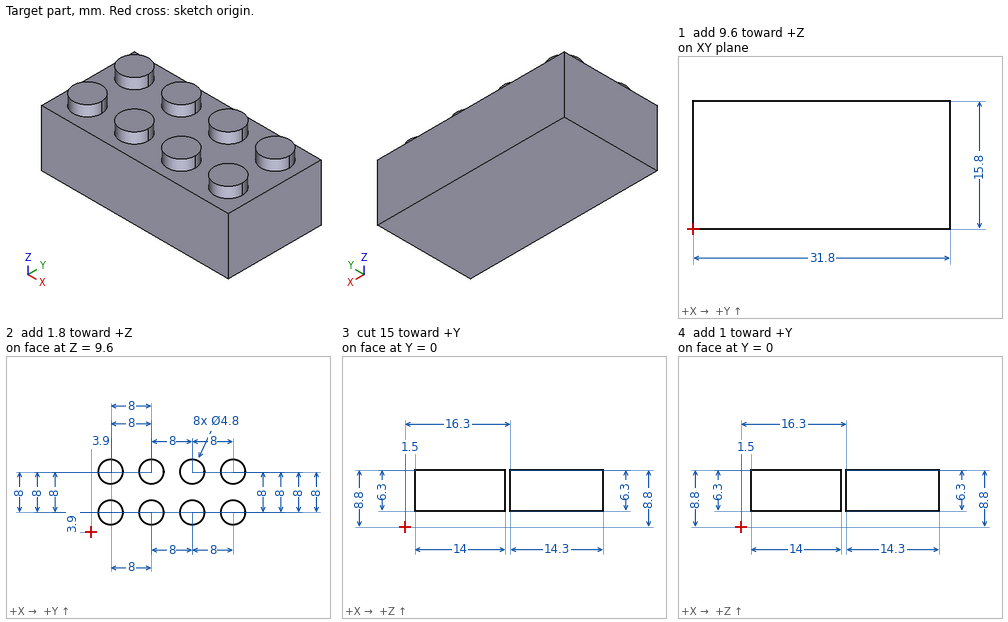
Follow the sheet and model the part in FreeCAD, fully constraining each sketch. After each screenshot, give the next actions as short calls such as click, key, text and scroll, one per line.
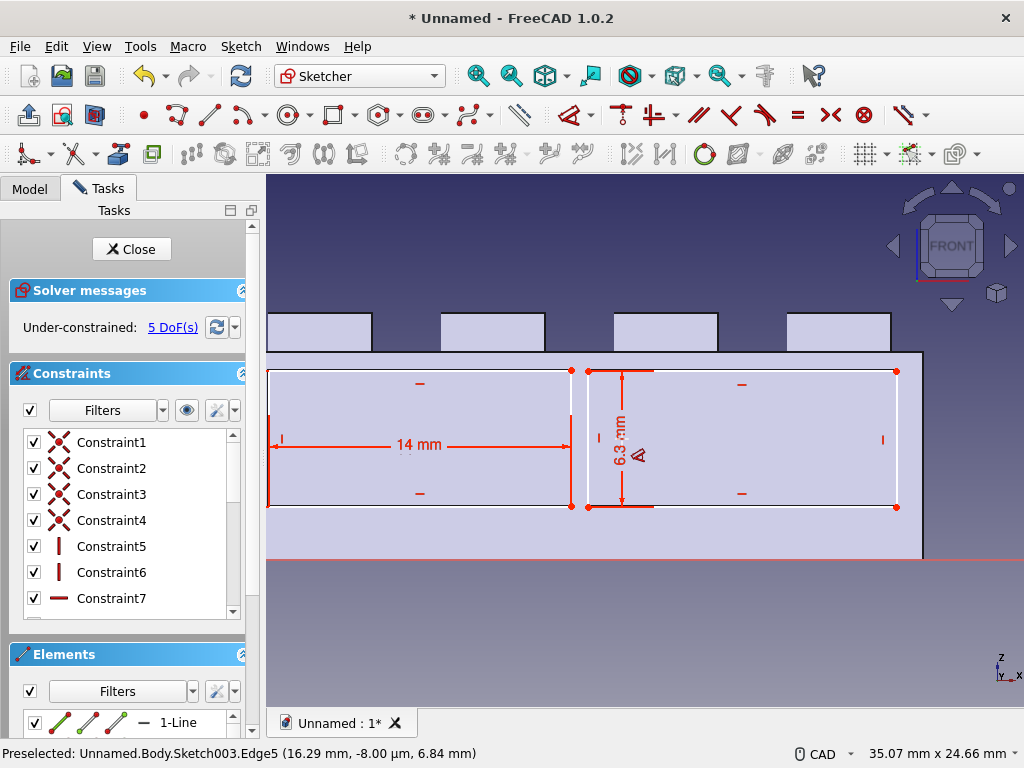
click(681, 507)
click(724, 541)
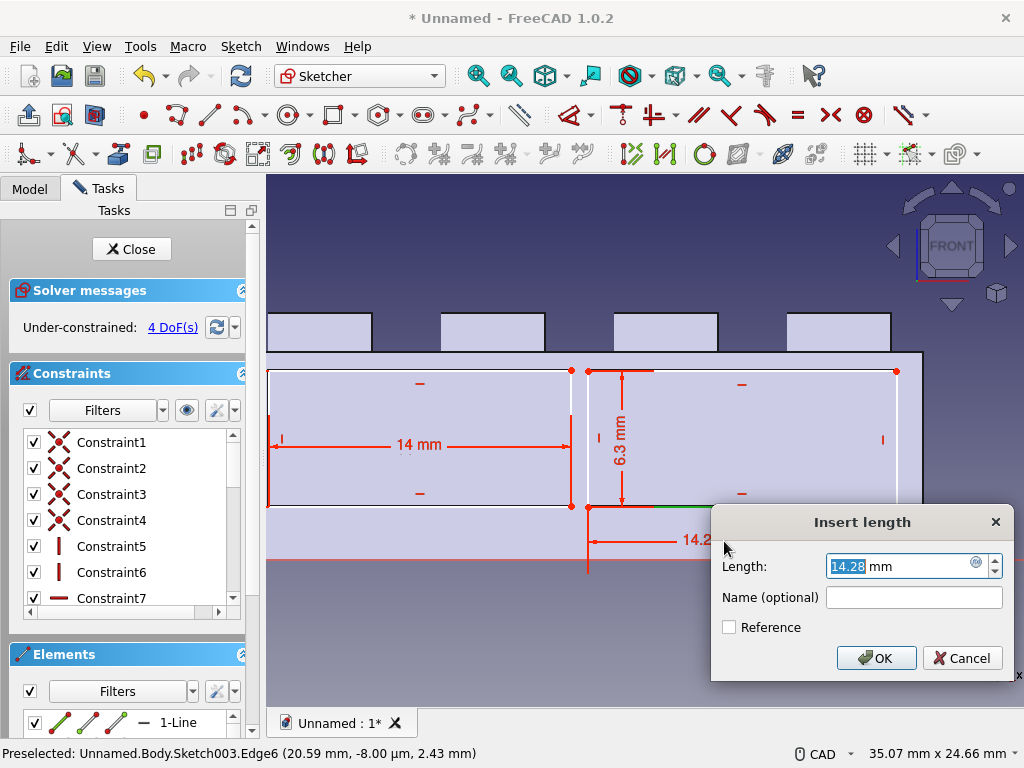
text(14.3)
key(Return)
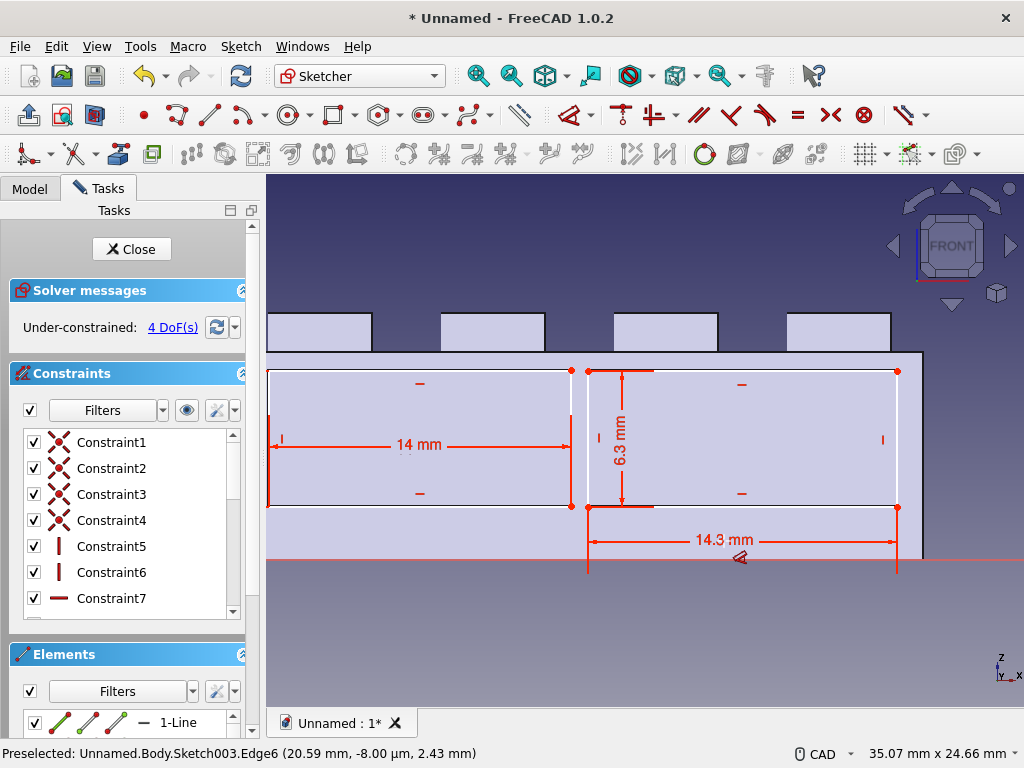
scroll(589, 411, down, 3)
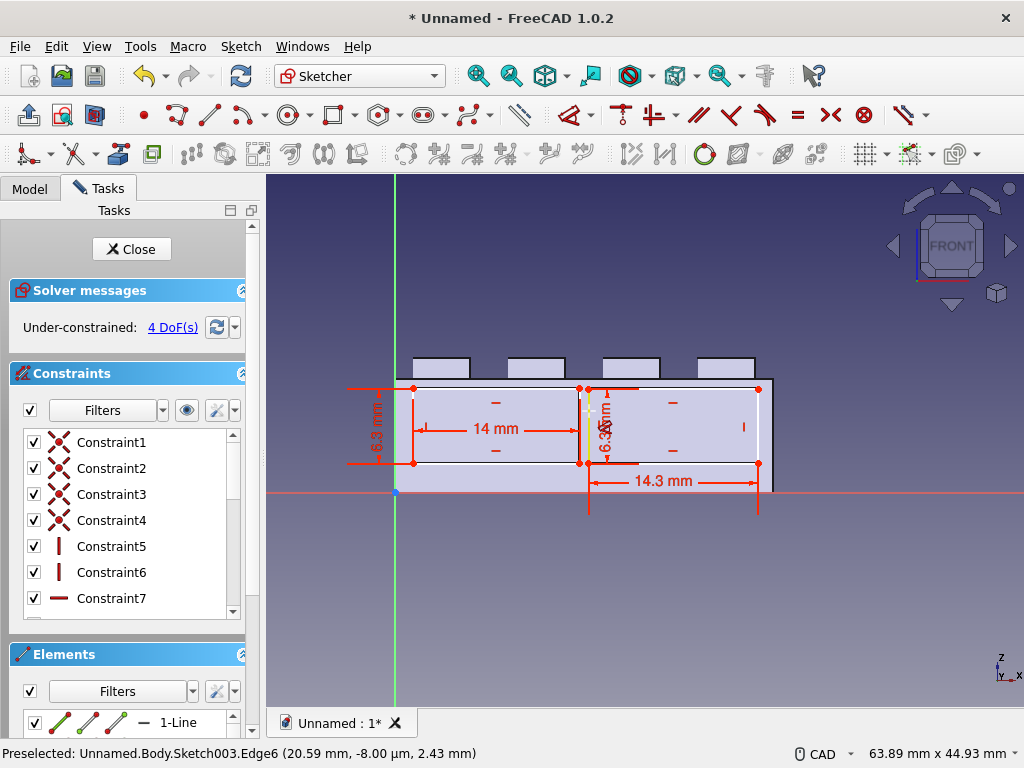
scroll(413, 389, up, 5)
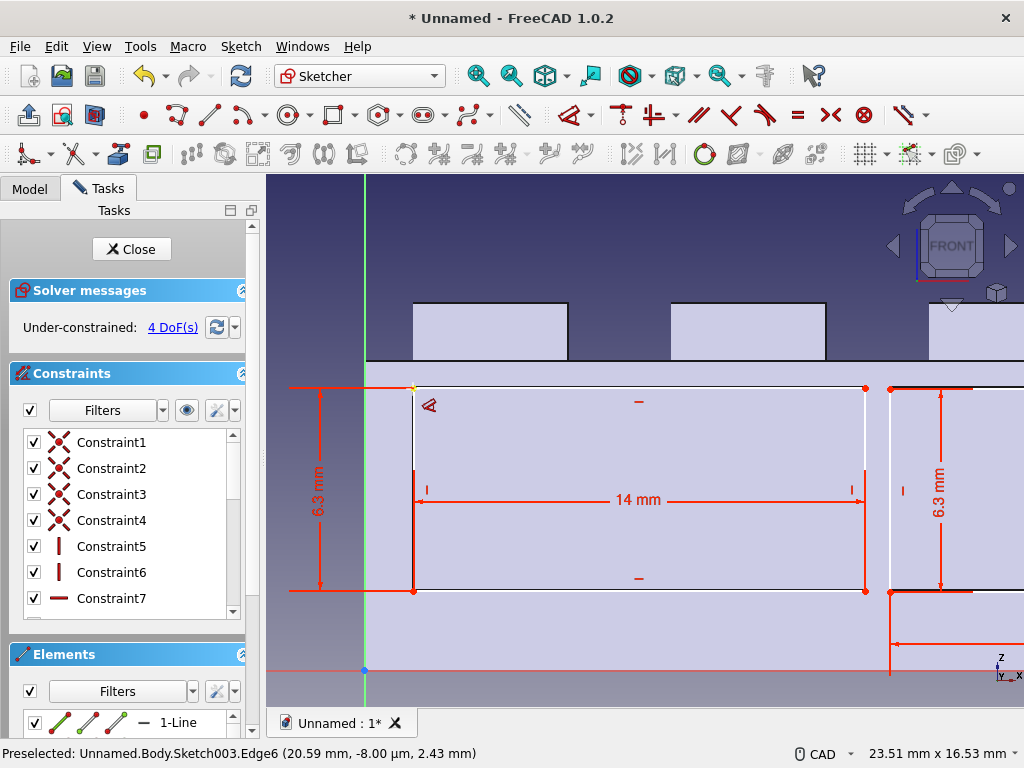
click(414, 388)
click(389, 354)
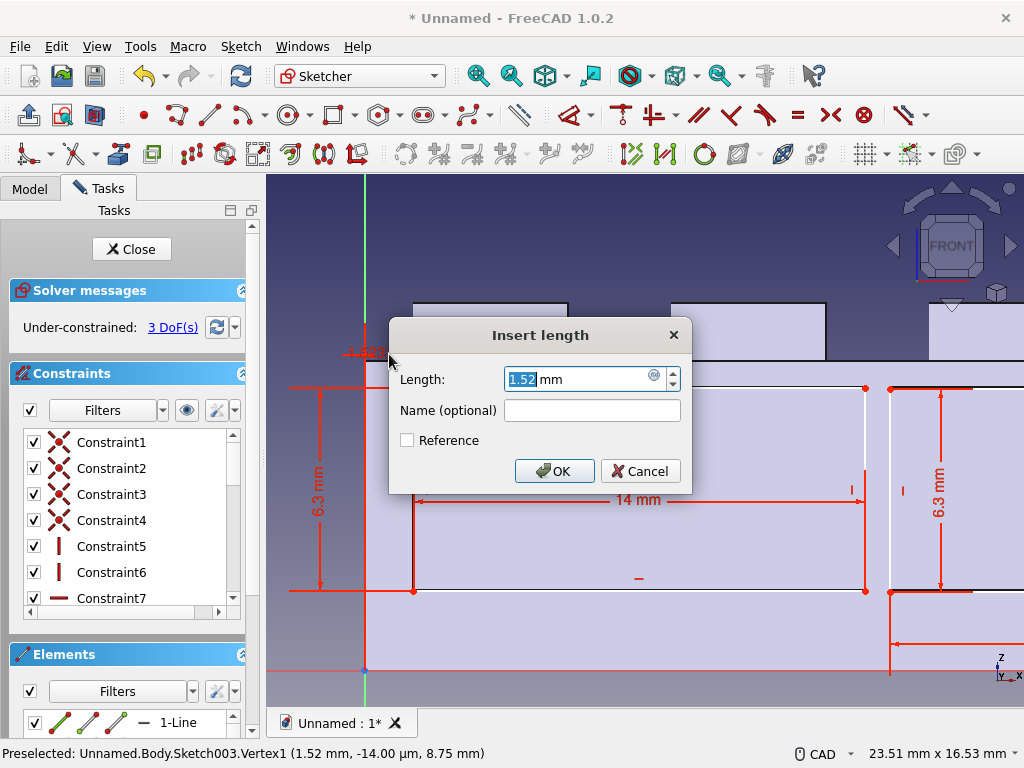
text(1.5)
key(Return)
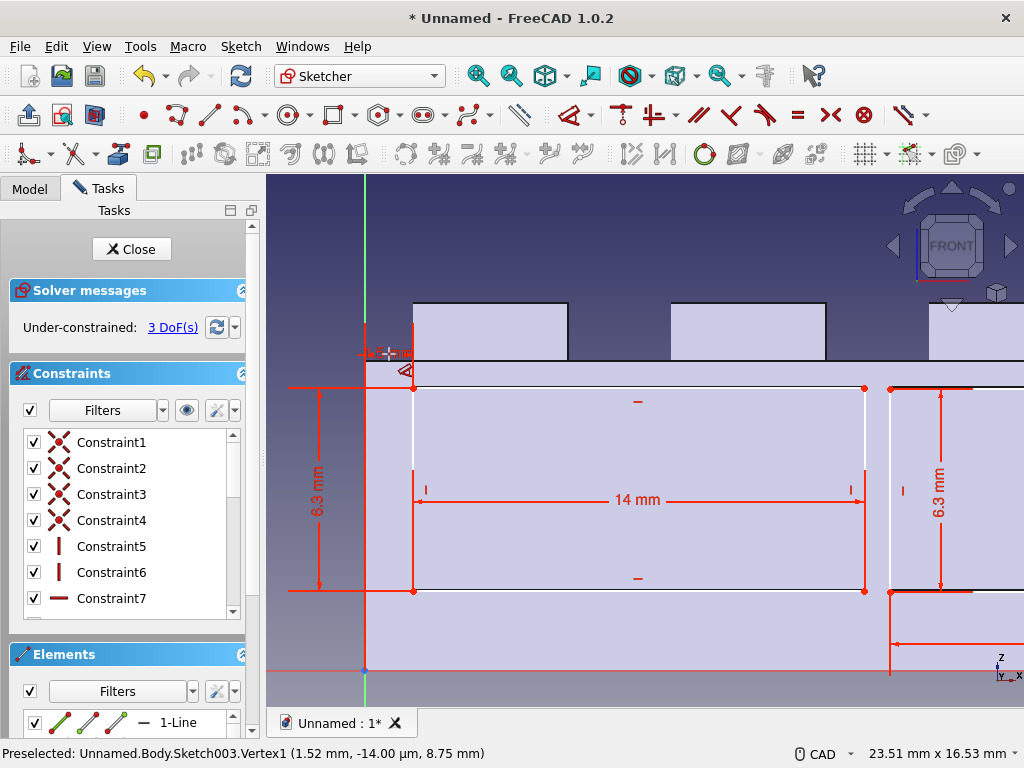
click(413, 388)
click(331, 529)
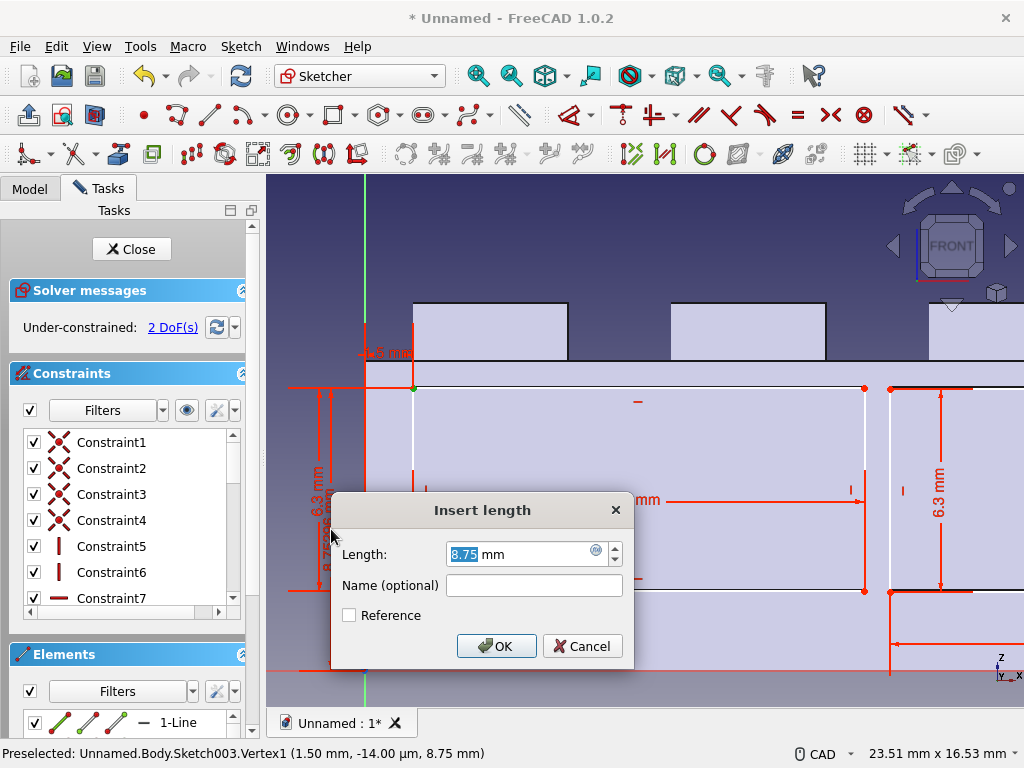
text(8.8)
key(Return)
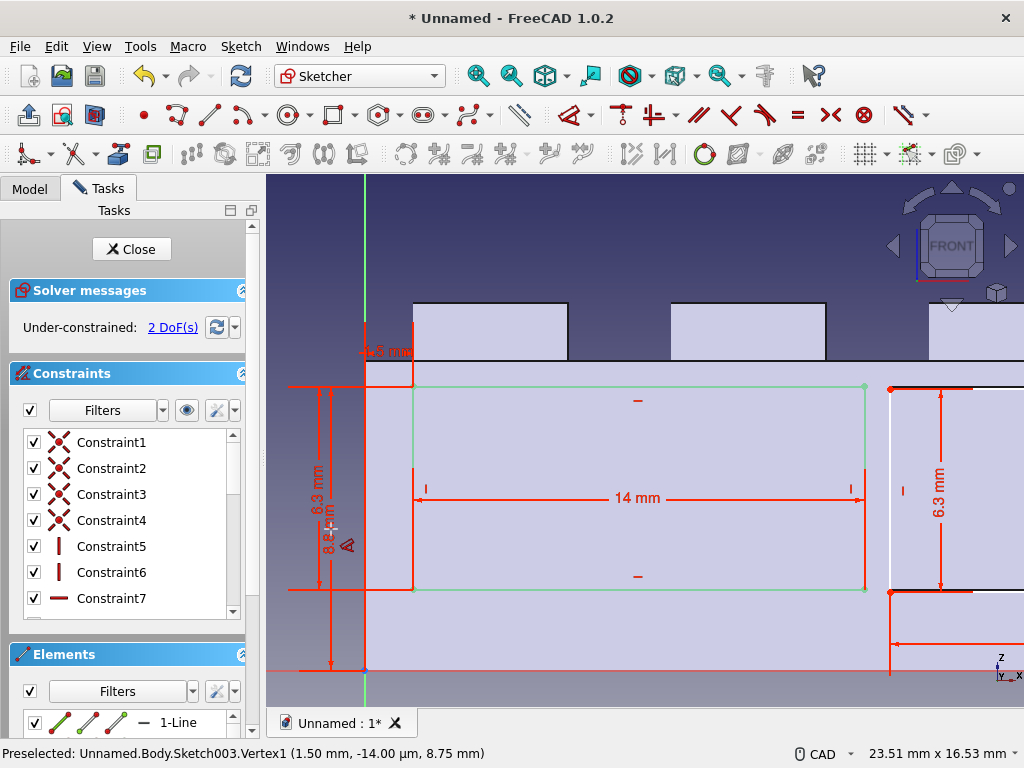
scroll(413, 389, down, 5)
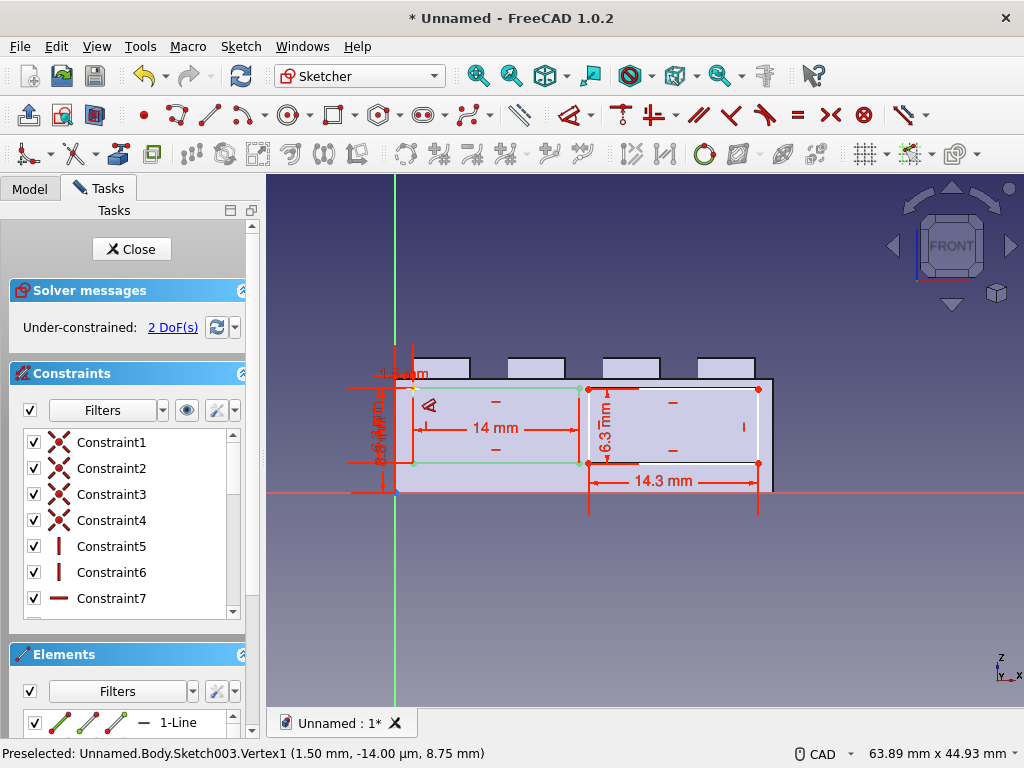
scroll(589, 389, up, 2)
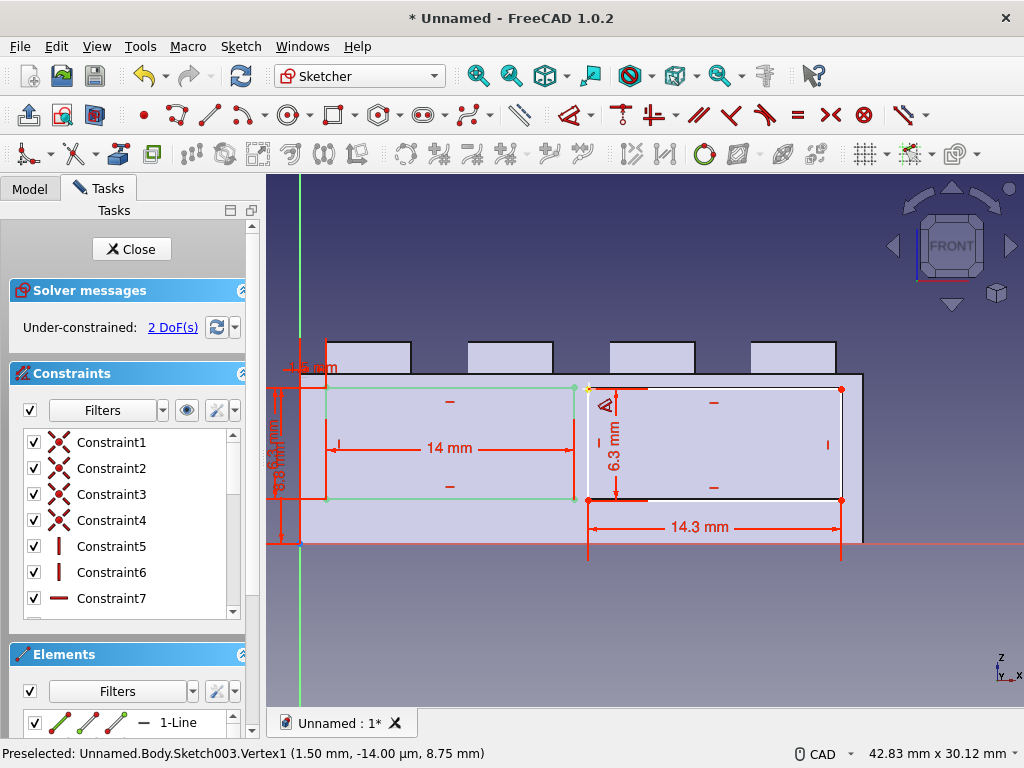
click(588, 389)
click(622, 466)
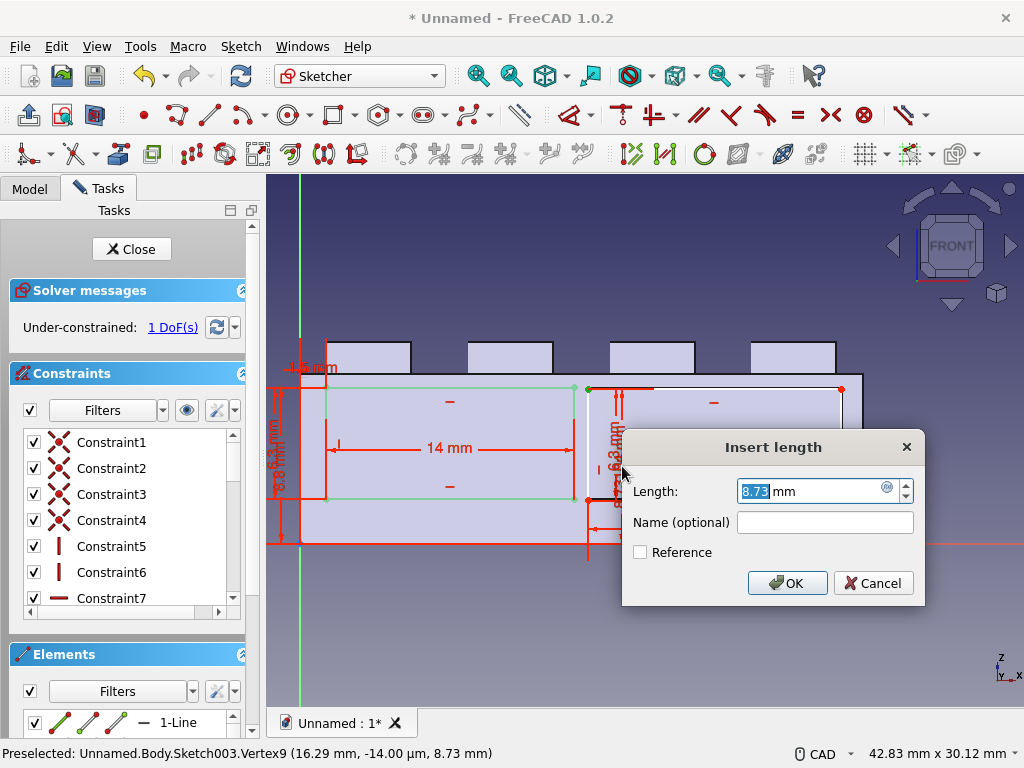
text(8.8)
key(Return)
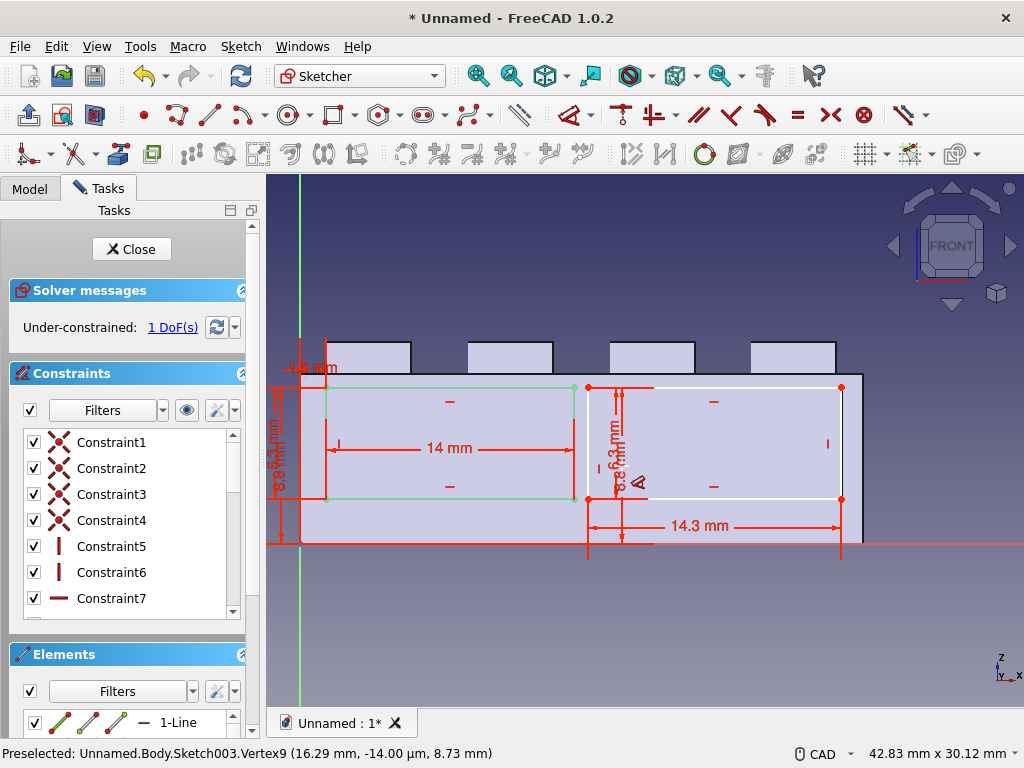
click(588, 388)
click(444, 578)